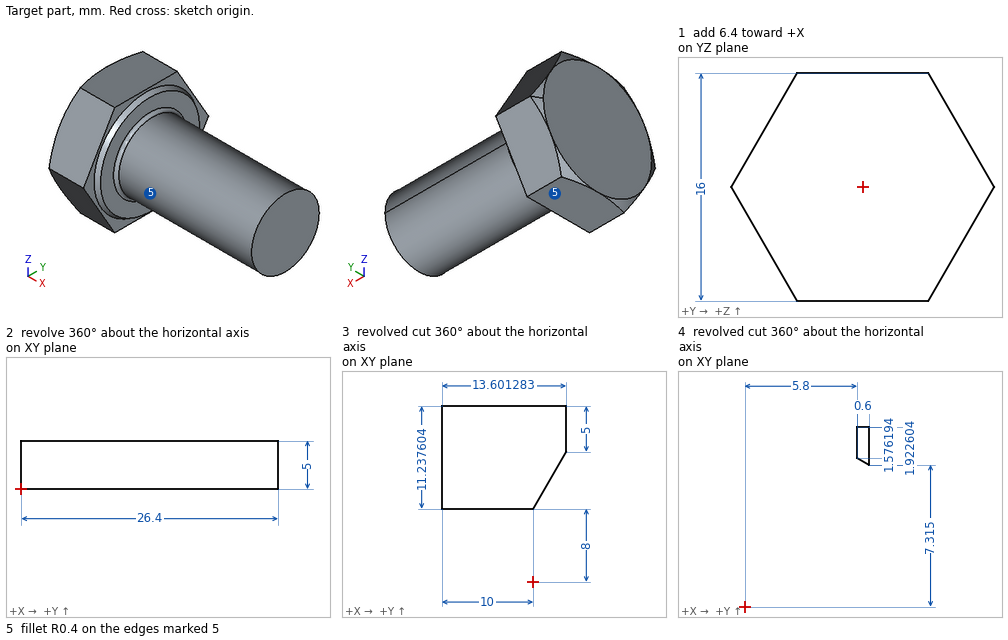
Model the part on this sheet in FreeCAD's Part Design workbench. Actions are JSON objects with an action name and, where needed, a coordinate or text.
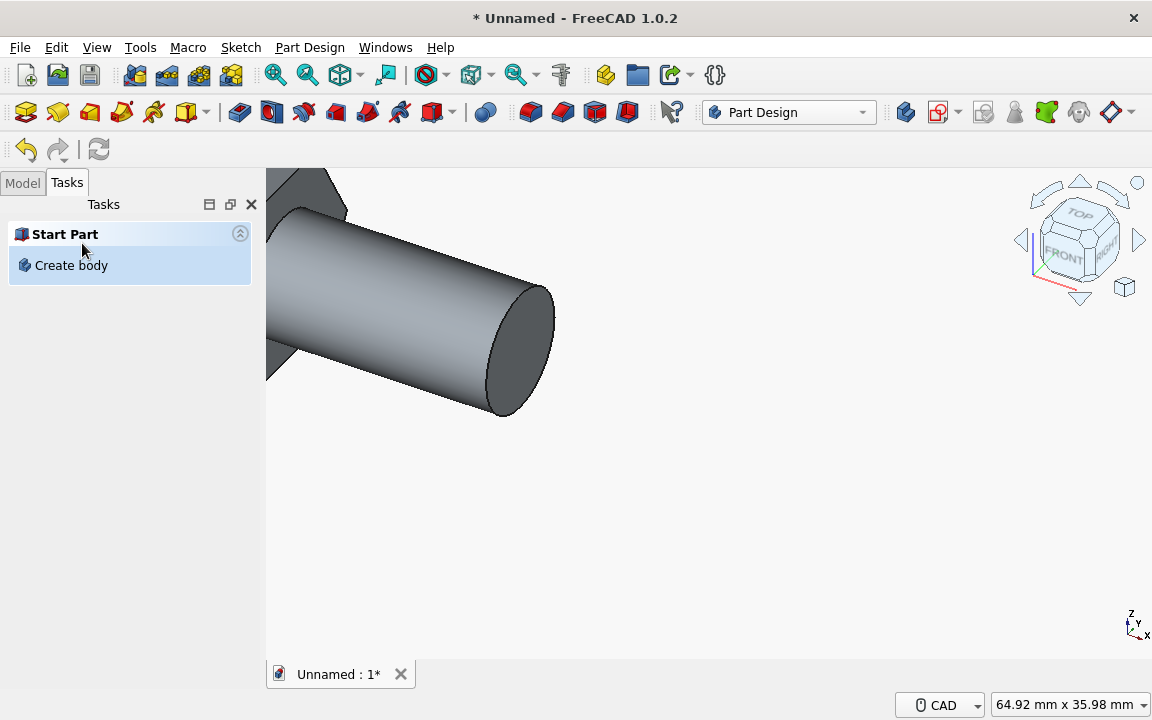
{"action": "left_click", "coordinate": [276, 76]}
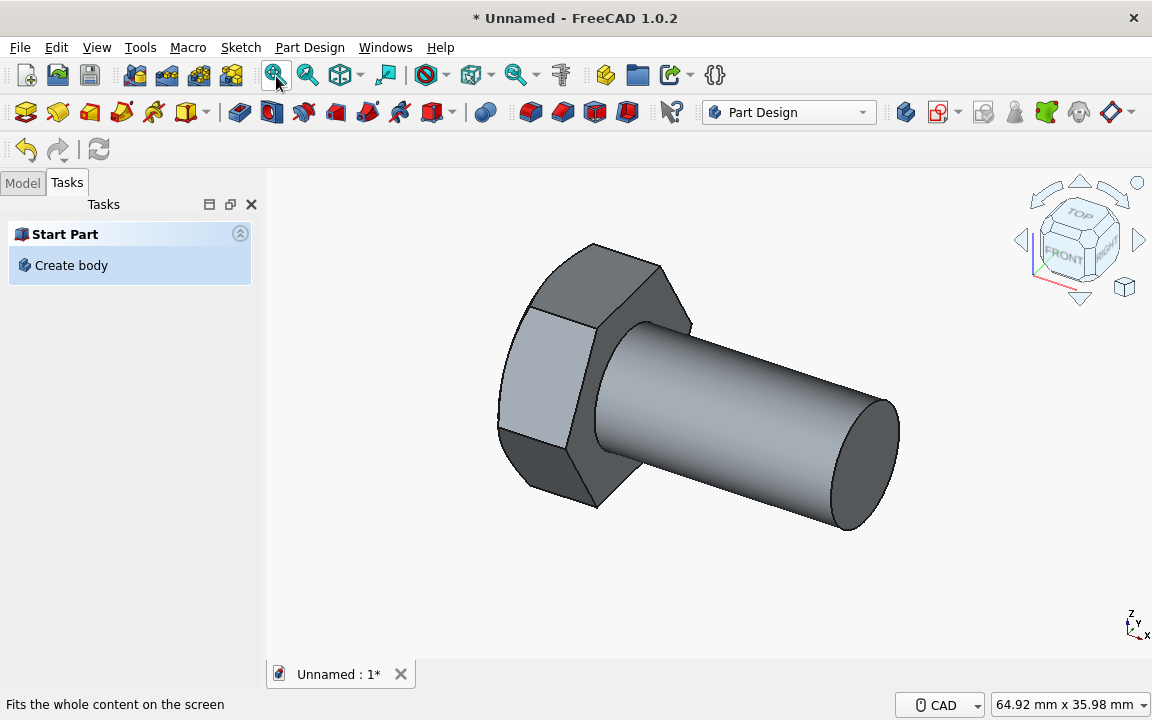
{"action": "left_click", "coordinate": [938, 112]}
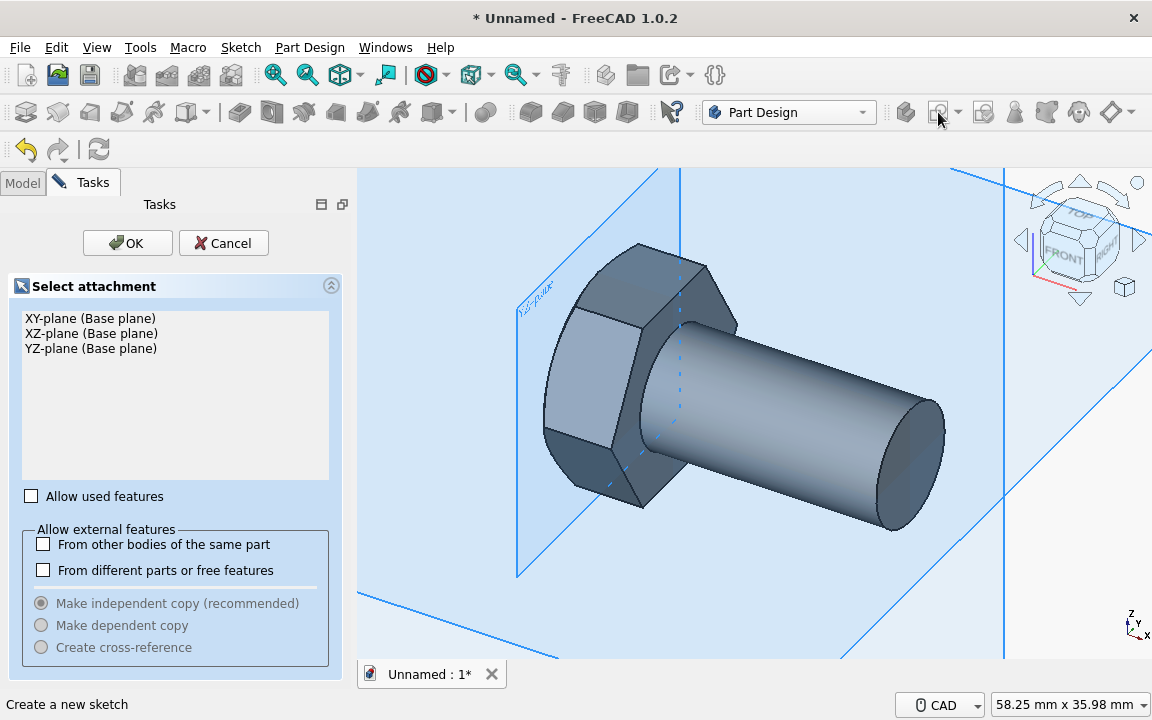
{"action": "left_click", "coordinate": [82, 318]}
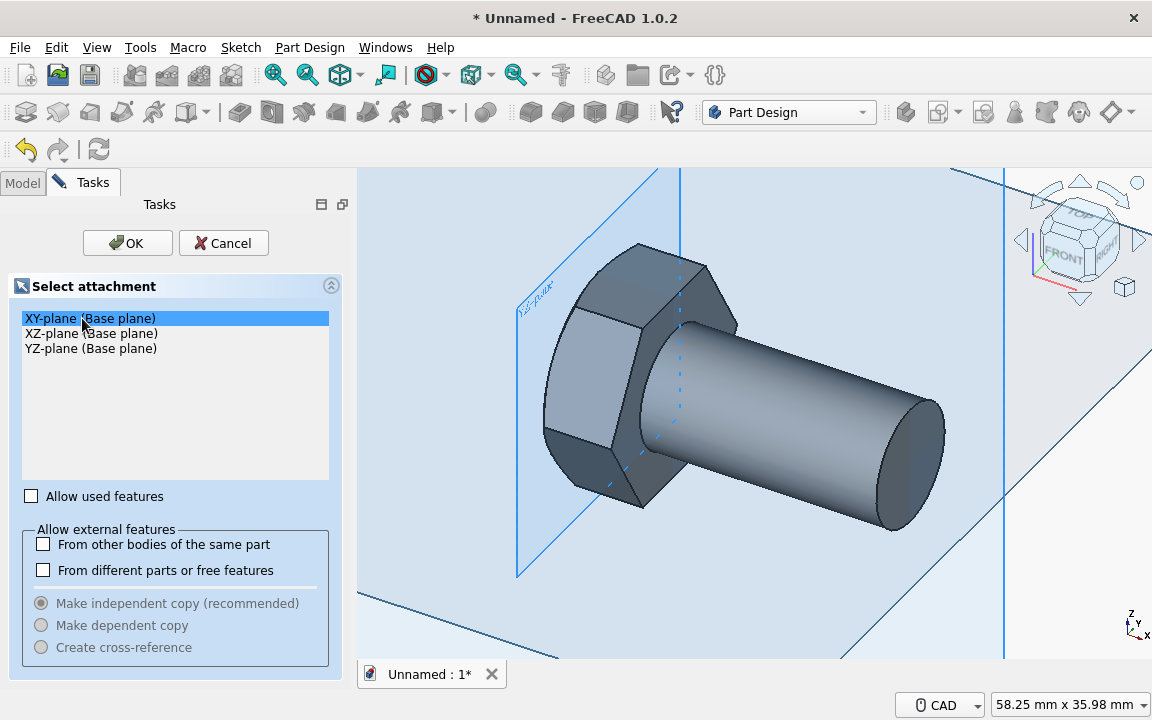
{"action": "left_click", "coordinate": [128, 243]}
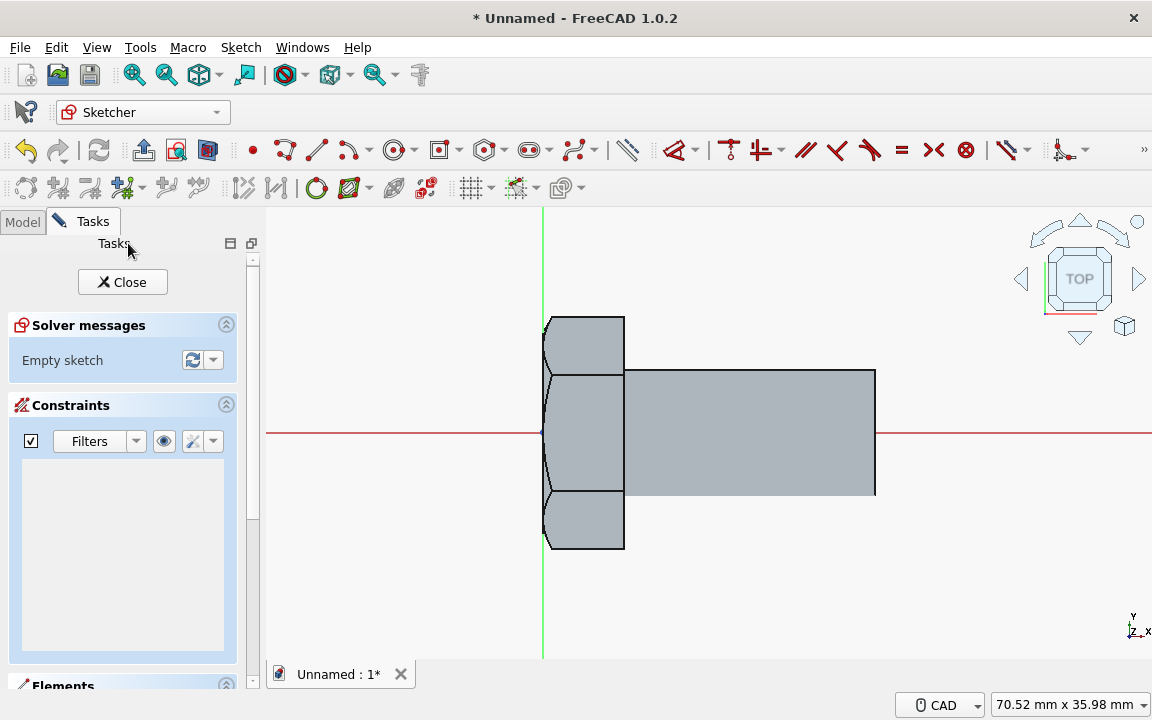
{"action": "left_click", "coordinate": [208, 150]}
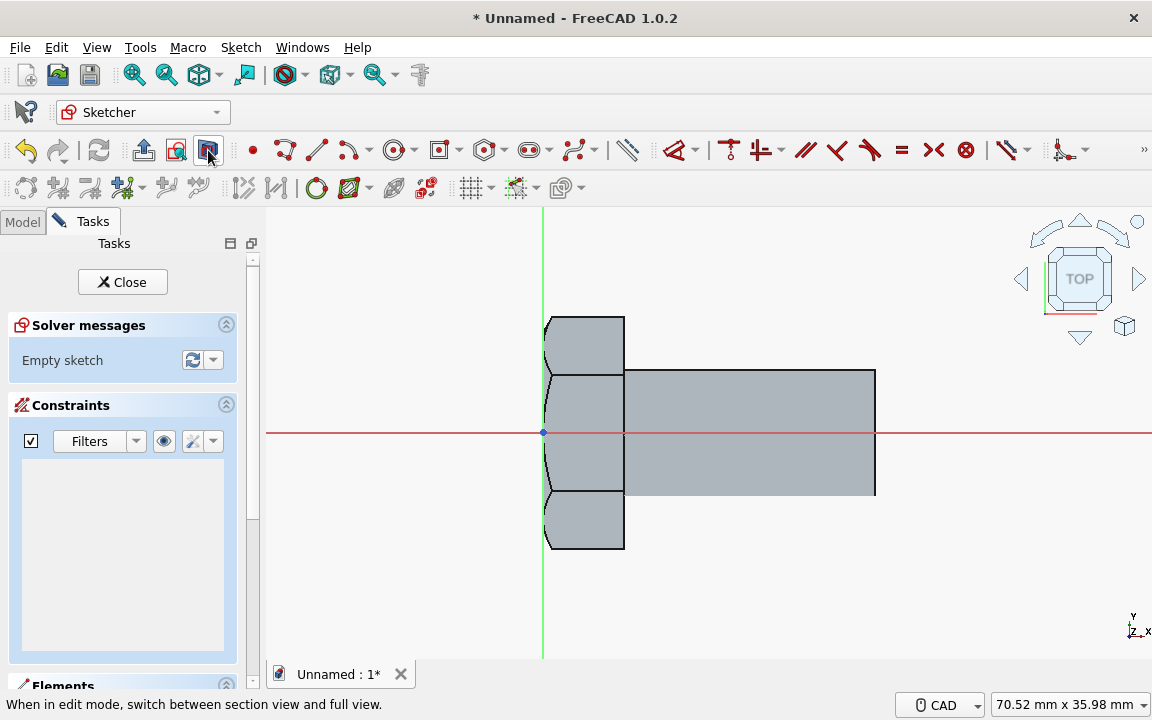
{"action": "scroll", "coordinate": [618, 319], "scroll_direction": "up", "scroll_amount": 12}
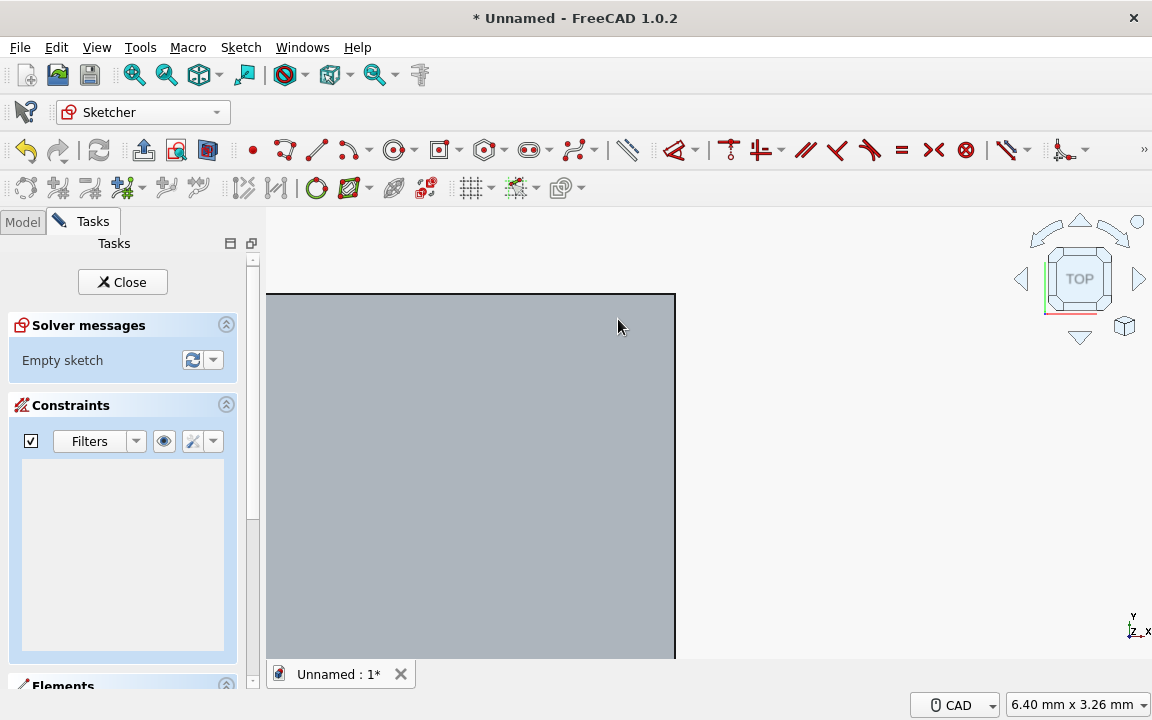
{"action": "left_click", "coordinate": [286, 150]}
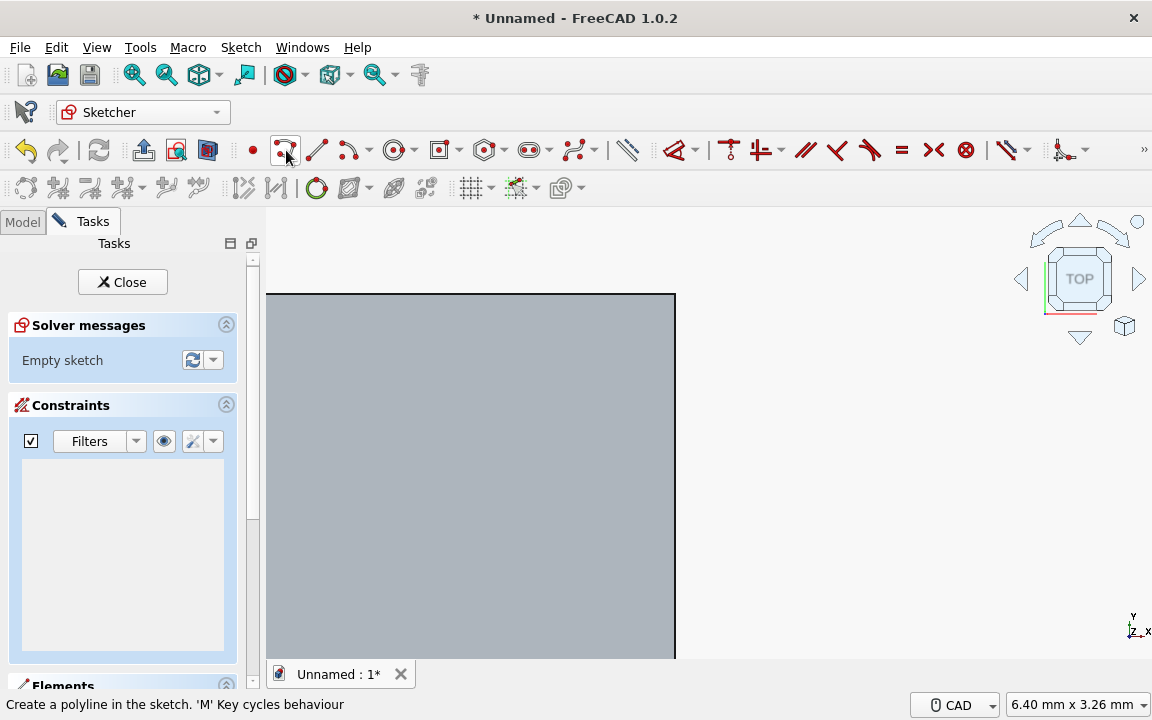
{"action": "left_click", "coordinate": [592, 512]}
{"action": "left_click", "coordinate": [675, 560]}
{"action": "left_click", "coordinate": [675, 294]}
{"action": "left_click", "coordinate": [592, 294]}
{"action": "left_click", "coordinate": [592, 513]}
{"action": "key", "text": "Escape"}
{"action": "key", "text": "Escape"}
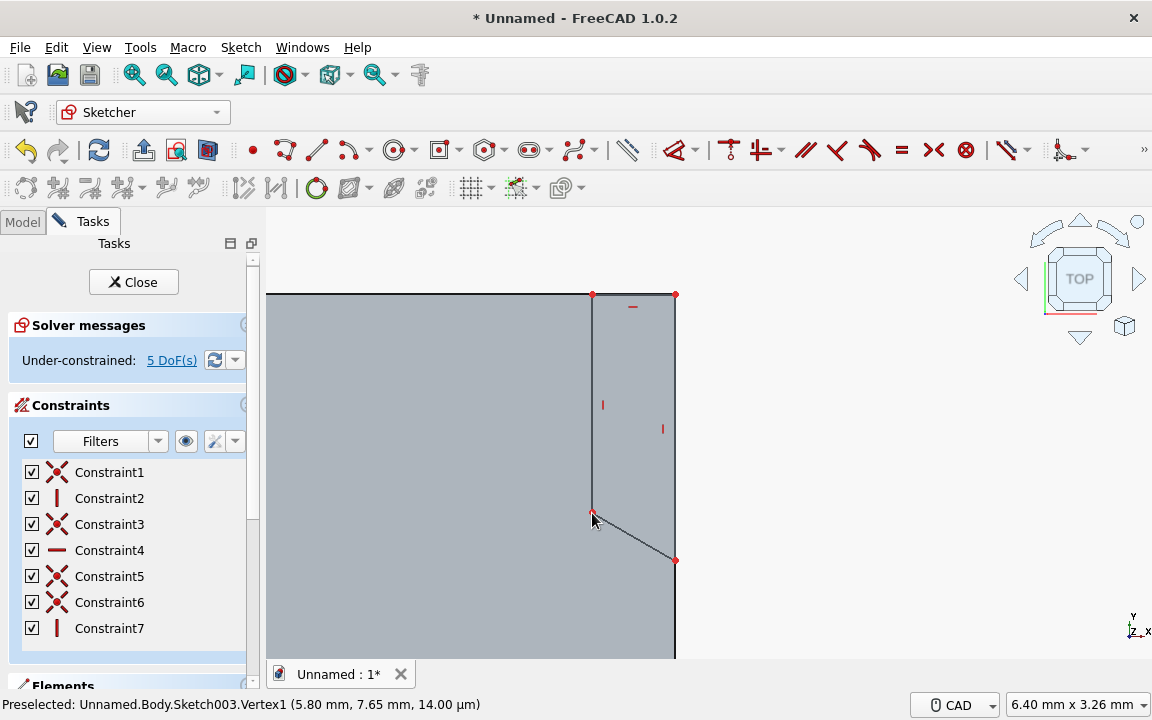
{"action": "left_click", "coordinate": [674, 150]}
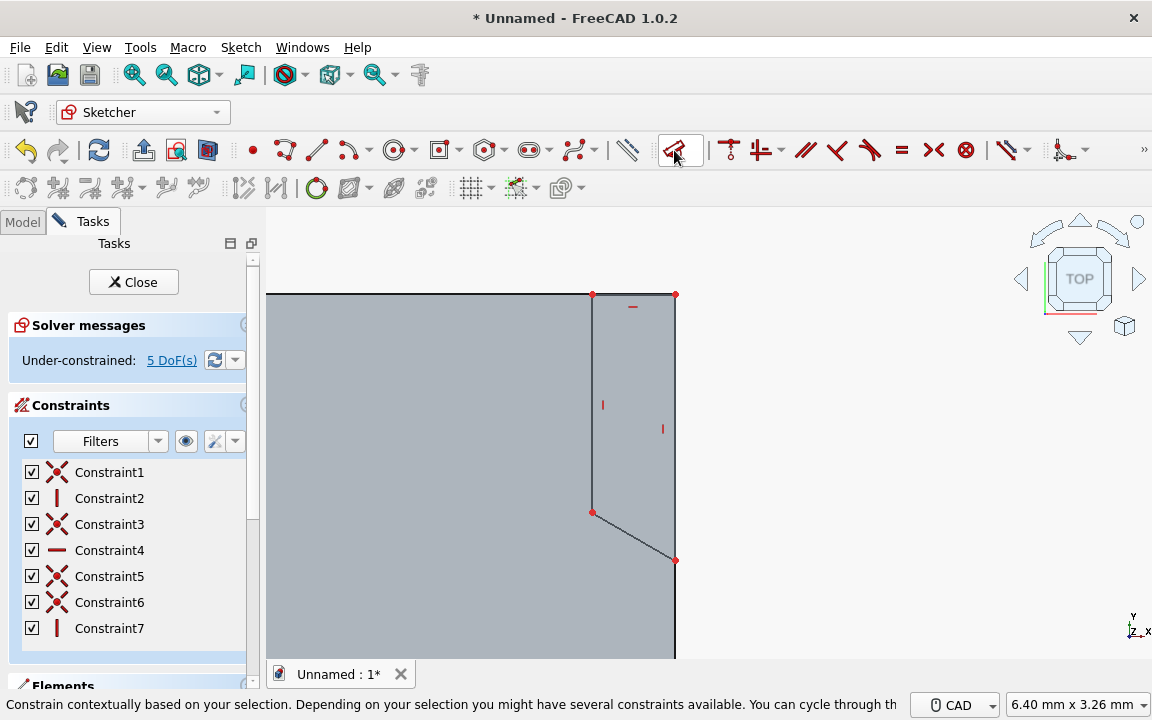
{"action": "left_click", "coordinate": [650, 295]}
{"action": "left_click", "coordinate": [634, 261]}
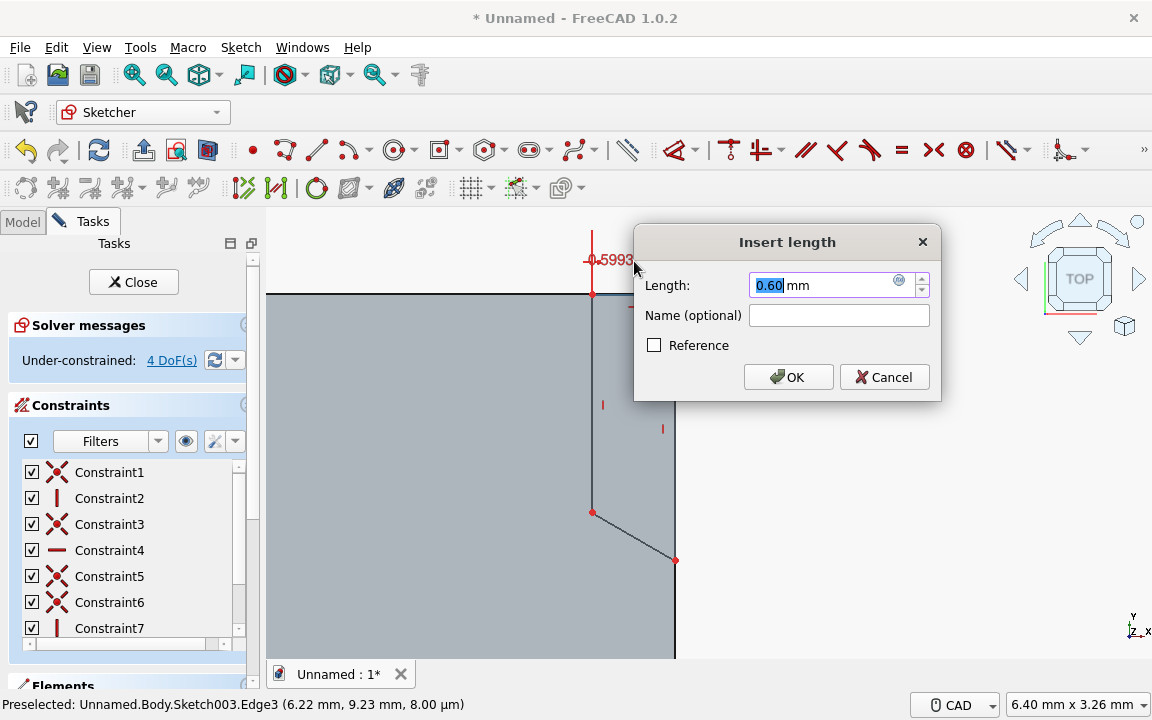
{"action": "type", "text": "0.6"}
{"action": "key", "text": "Return"}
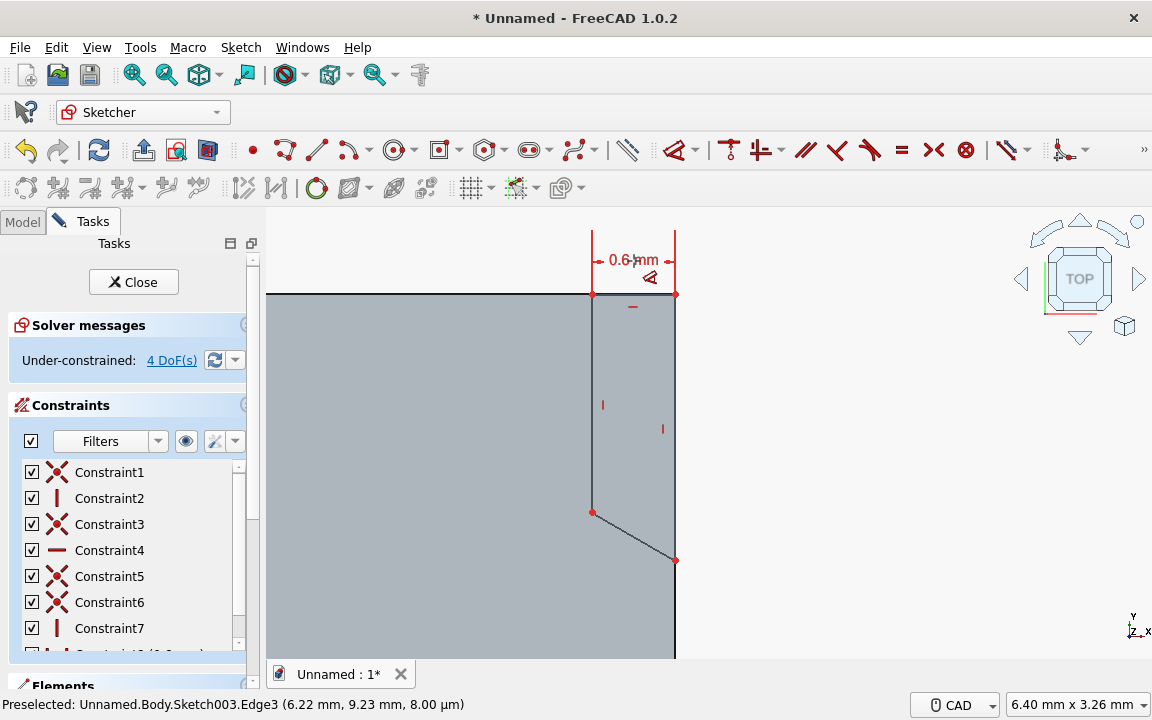
{"action": "left_click", "coordinate": [592, 513]}
{"action": "left_click", "coordinate": [443, 479]}